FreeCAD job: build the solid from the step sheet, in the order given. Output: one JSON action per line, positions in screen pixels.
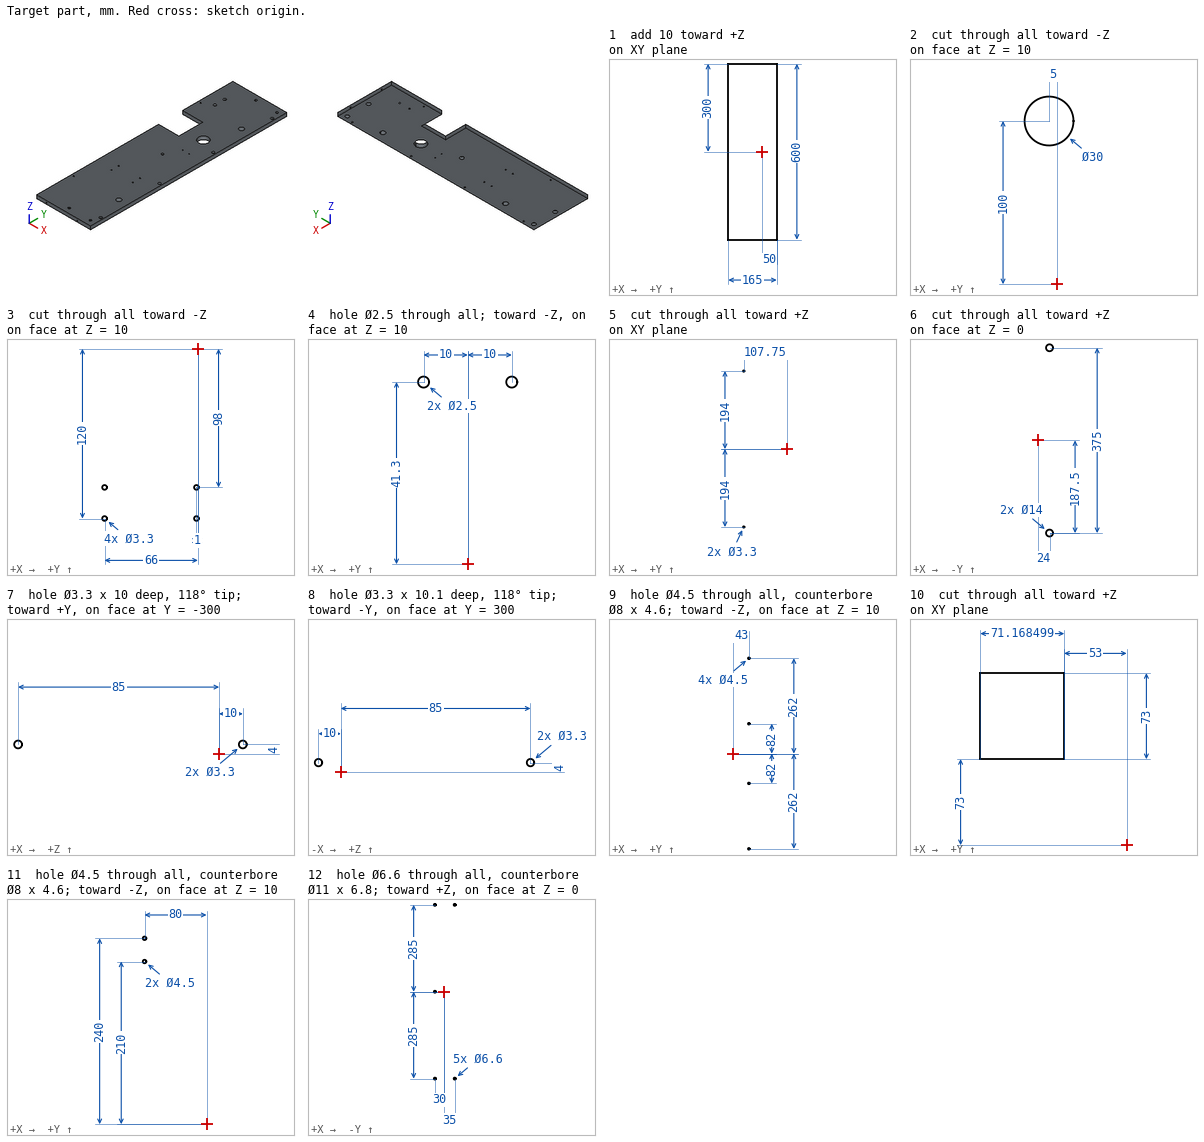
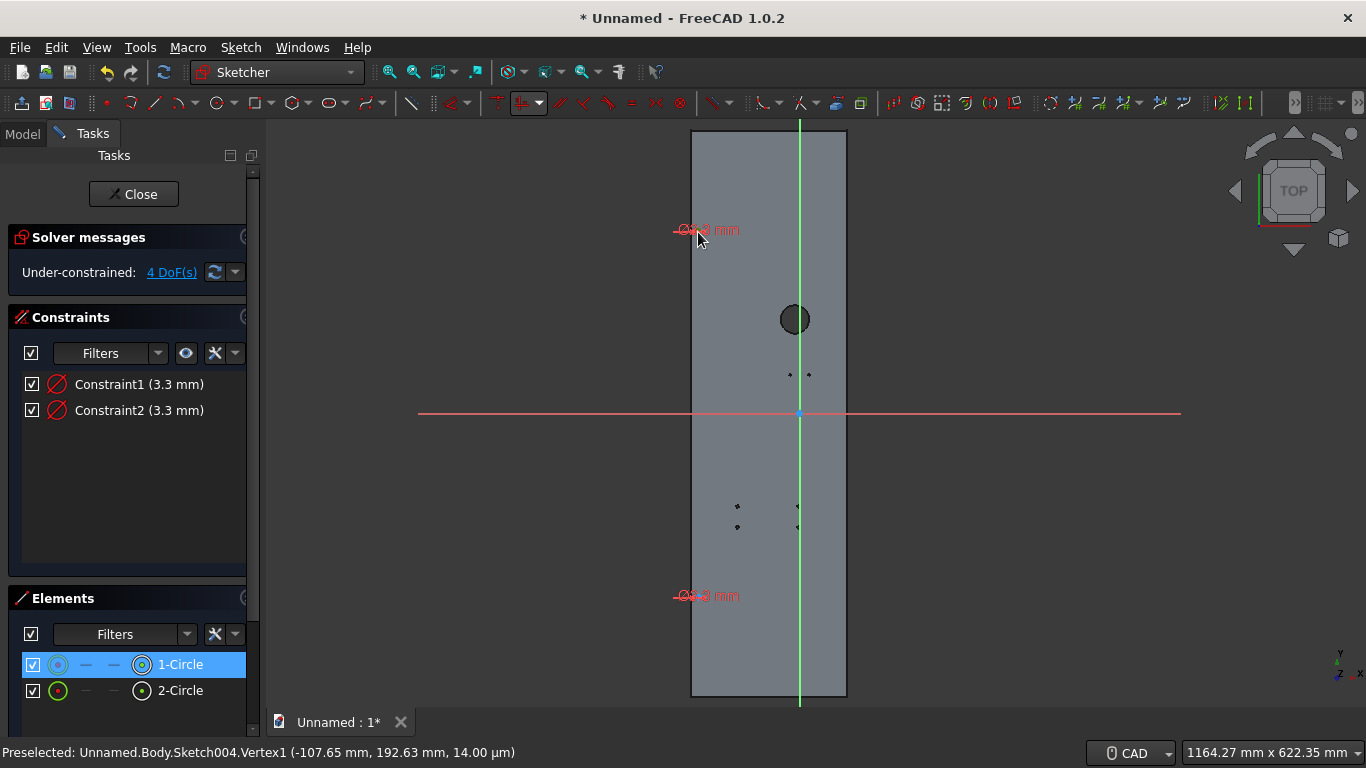
{"action": "left_click", "coordinate": [698, 598]}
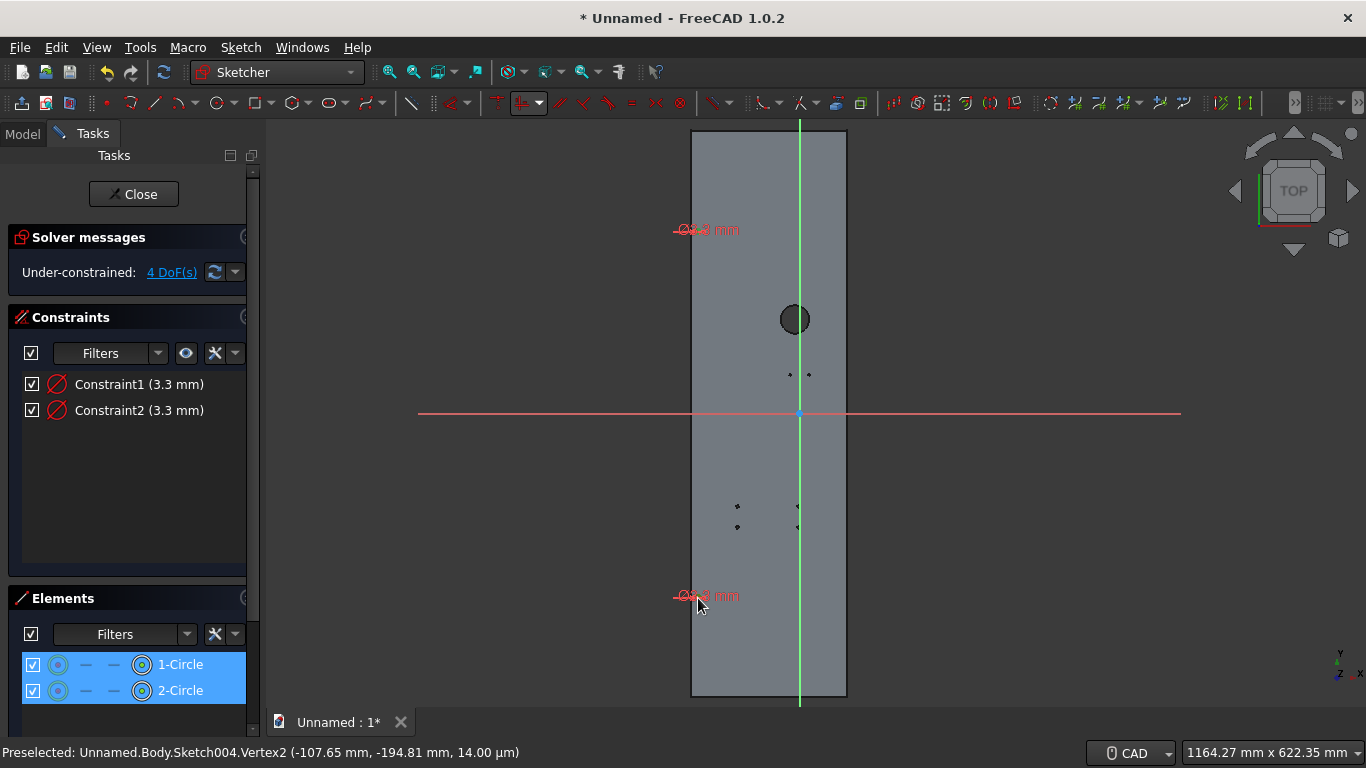
{"action": "key", "text": "v"}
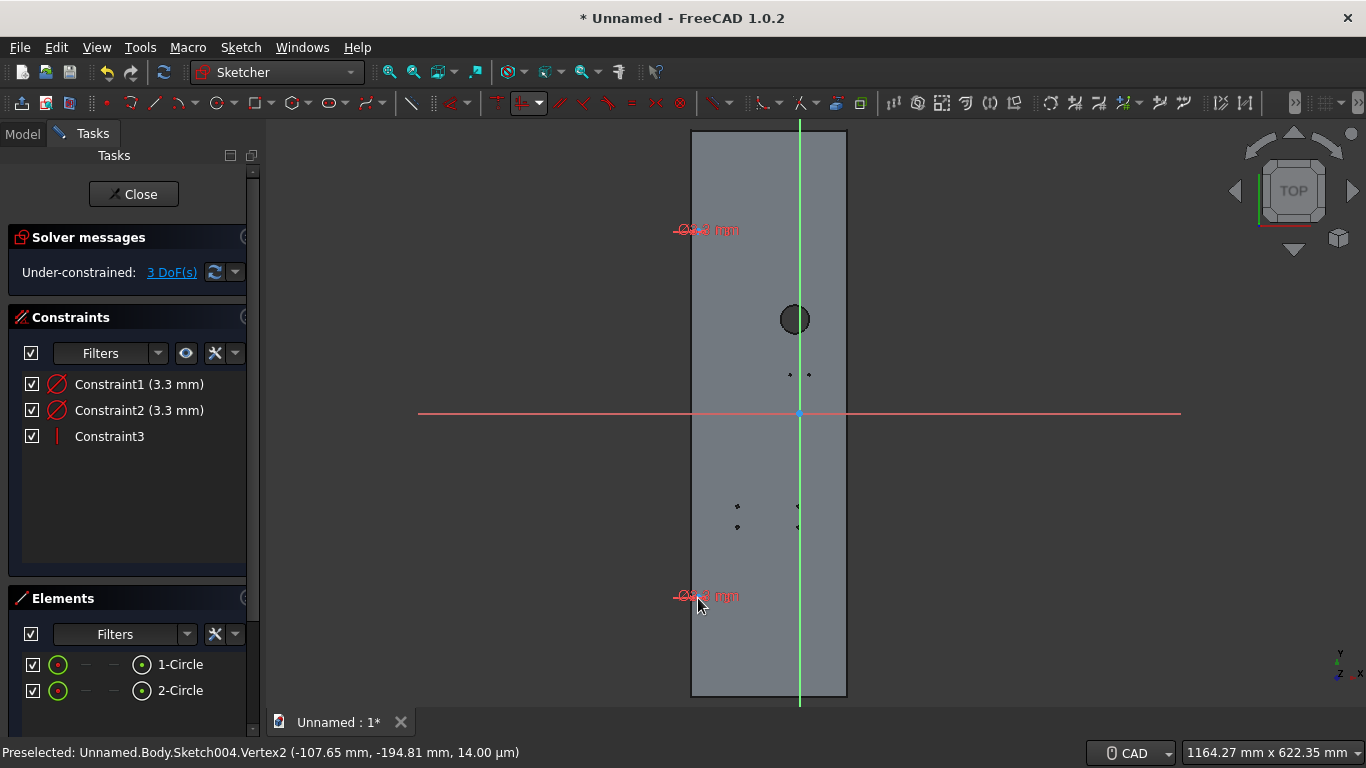
{"action": "left_click", "coordinate": [450, 104]}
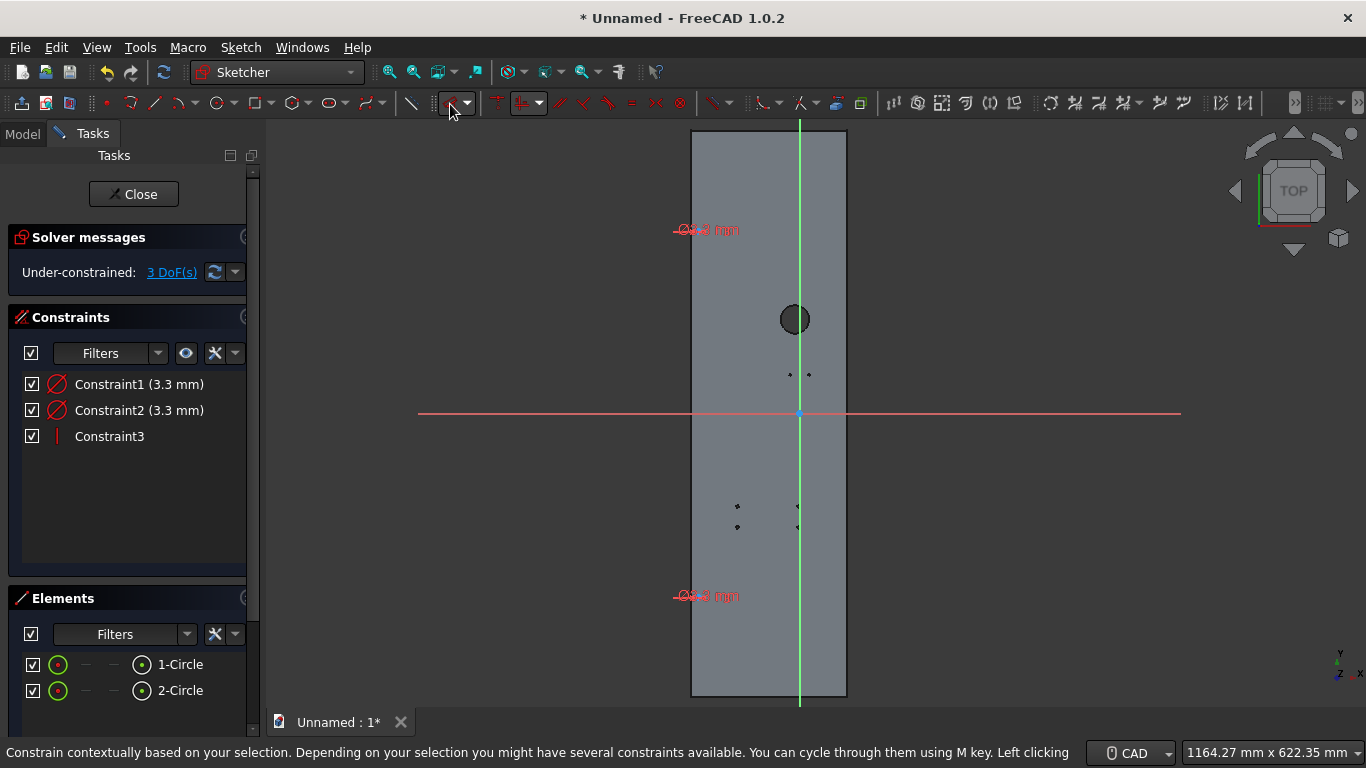
{"action": "left_click", "coordinate": [698, 232]}
{"action": "left_click", "coordinate": [834, 323]}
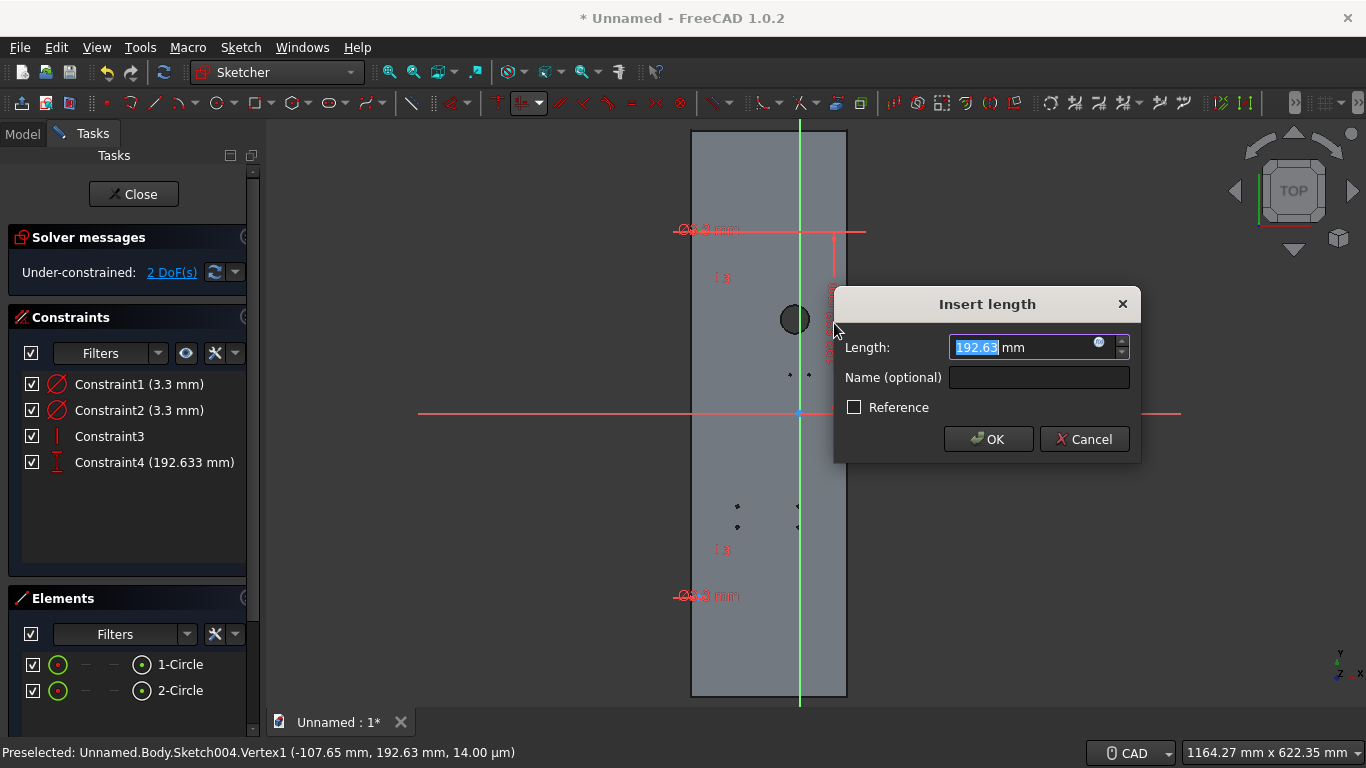
{"action": "type", "text": "194"}
{"action": "key", "text": "Return"}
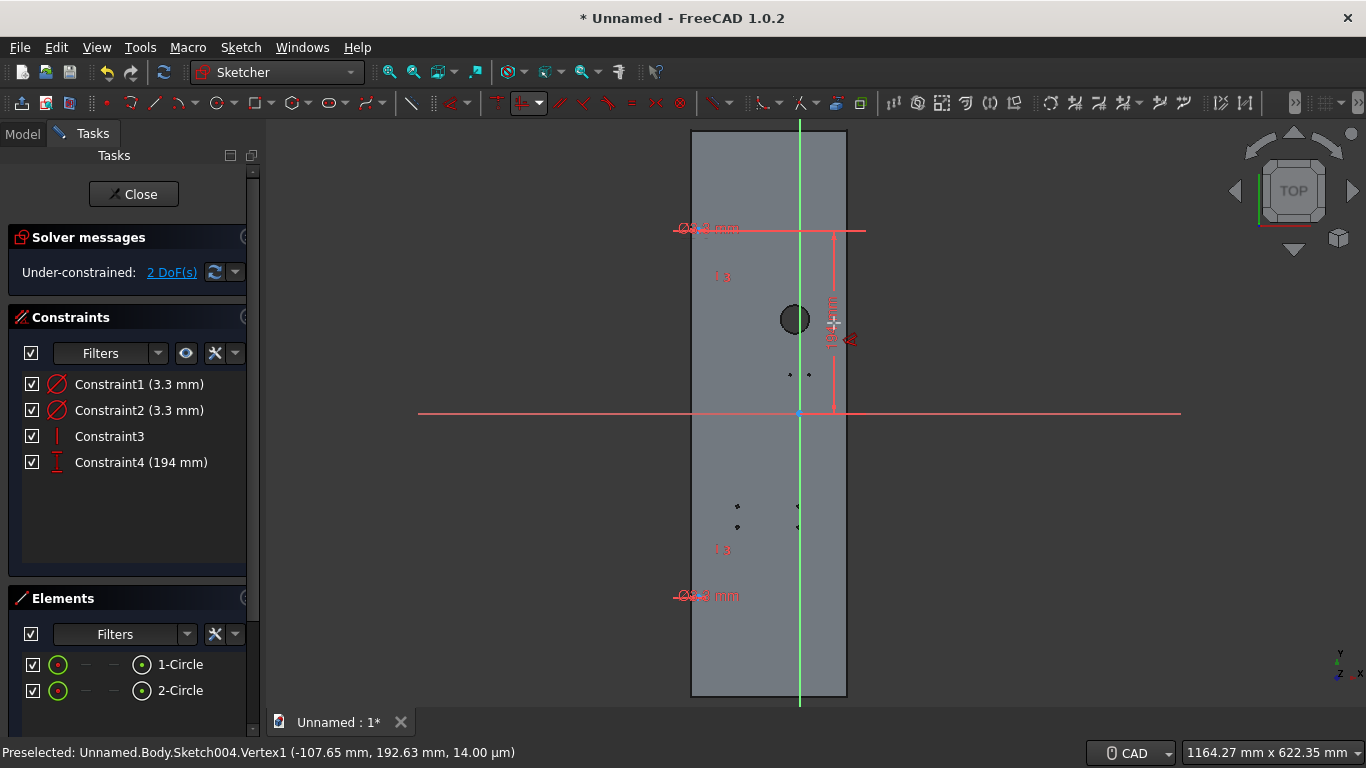
{"action": "left_click", "coordinate": [698, 598]}
{"action": "left_click", "coordinate": [834, 506]}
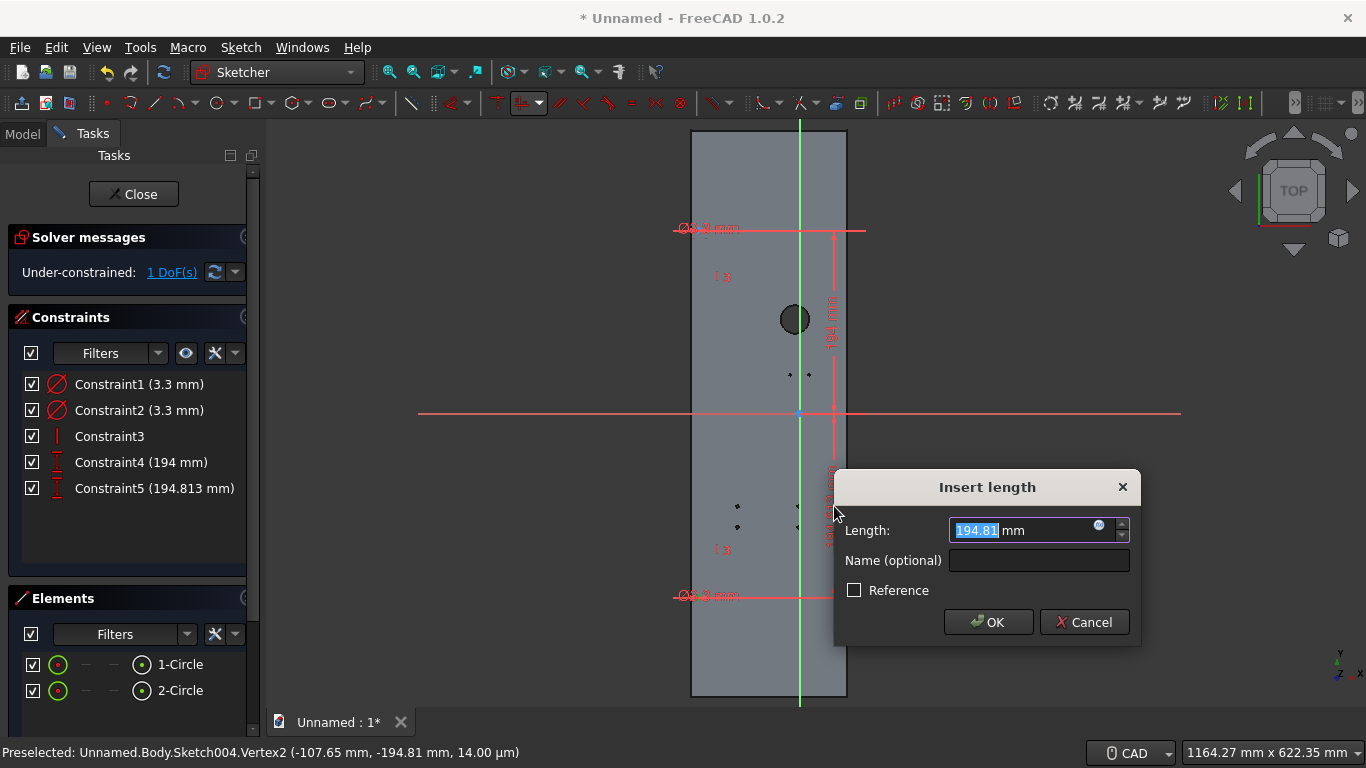
{"action": "type", "text": "194"}
{"action": "key", "text": "Return"}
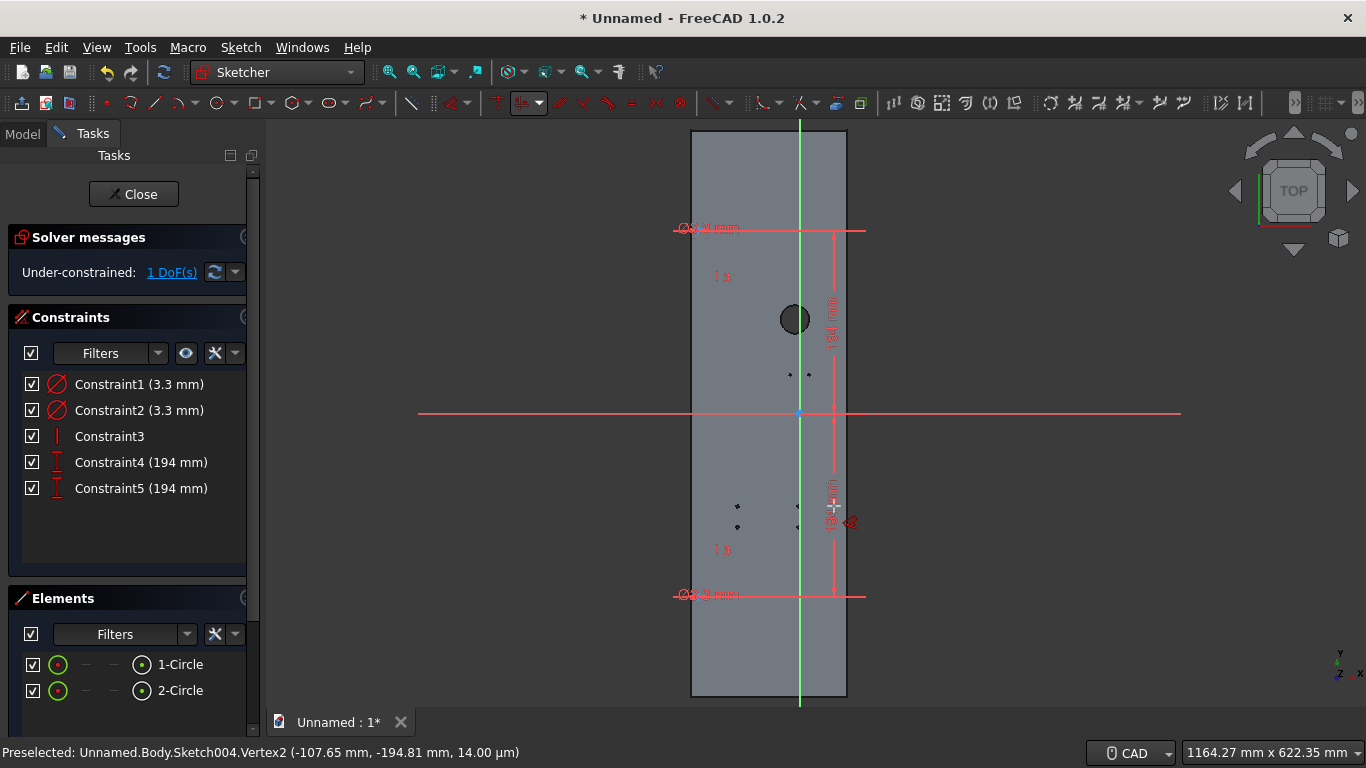
{"action": "left_click", "coordinate": [698, 231]}
{"action": "left_click", "coordinate": [749, 197]}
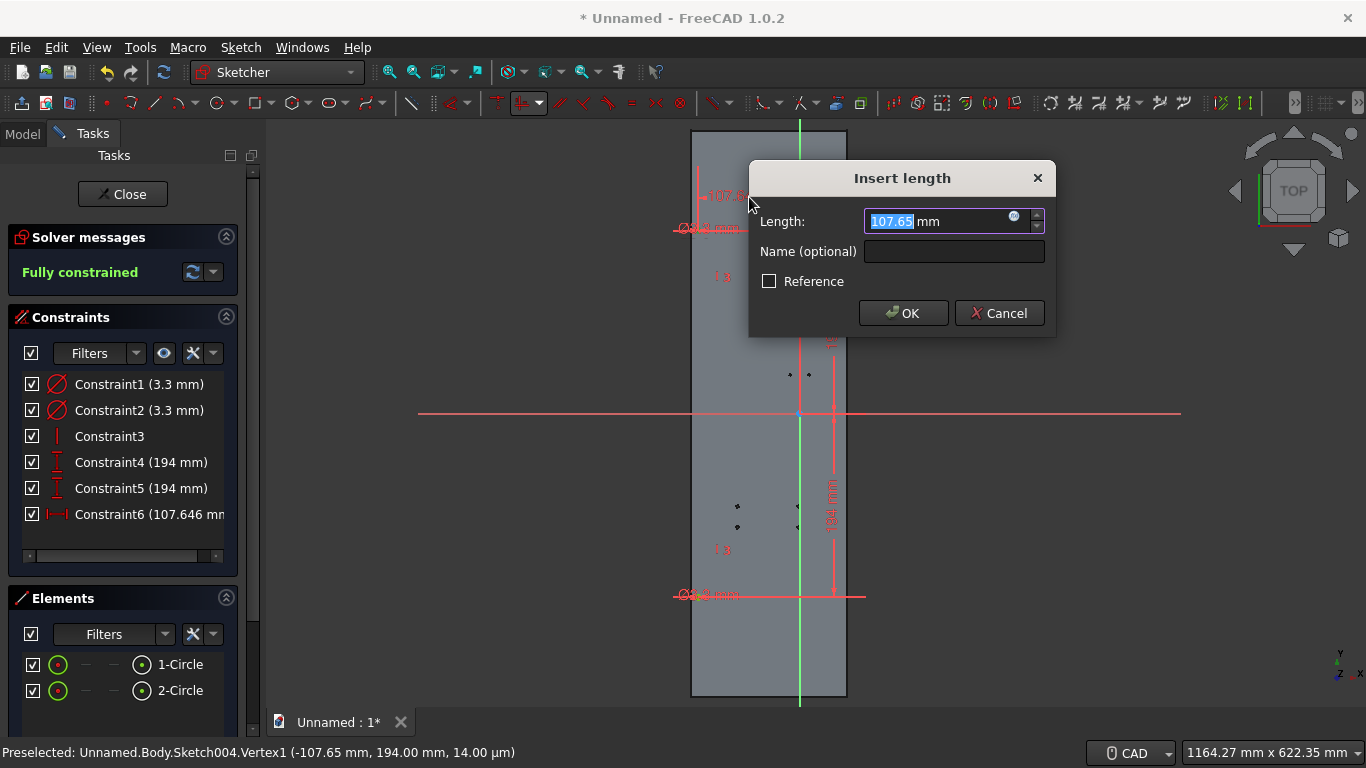
{"action": "type", "text": "107.75"}
{"action": "key", "text": "Return"}
{"action": "key", "text": "Escape"}